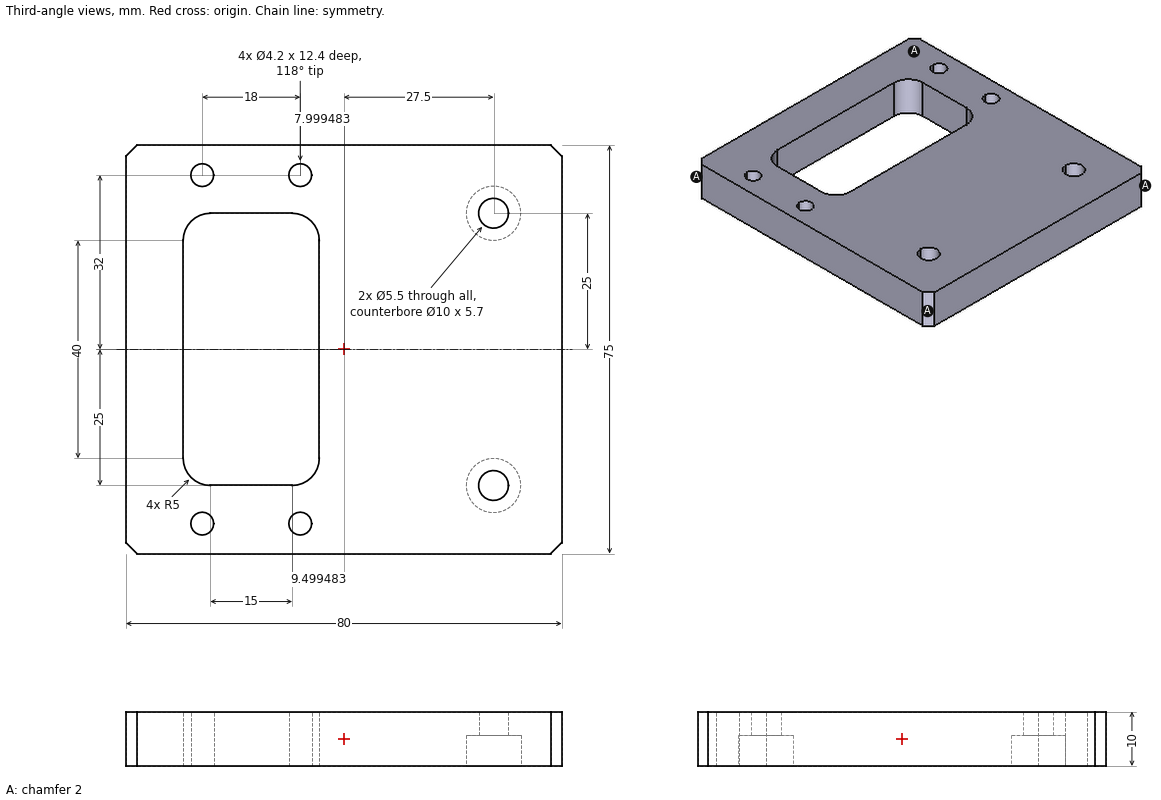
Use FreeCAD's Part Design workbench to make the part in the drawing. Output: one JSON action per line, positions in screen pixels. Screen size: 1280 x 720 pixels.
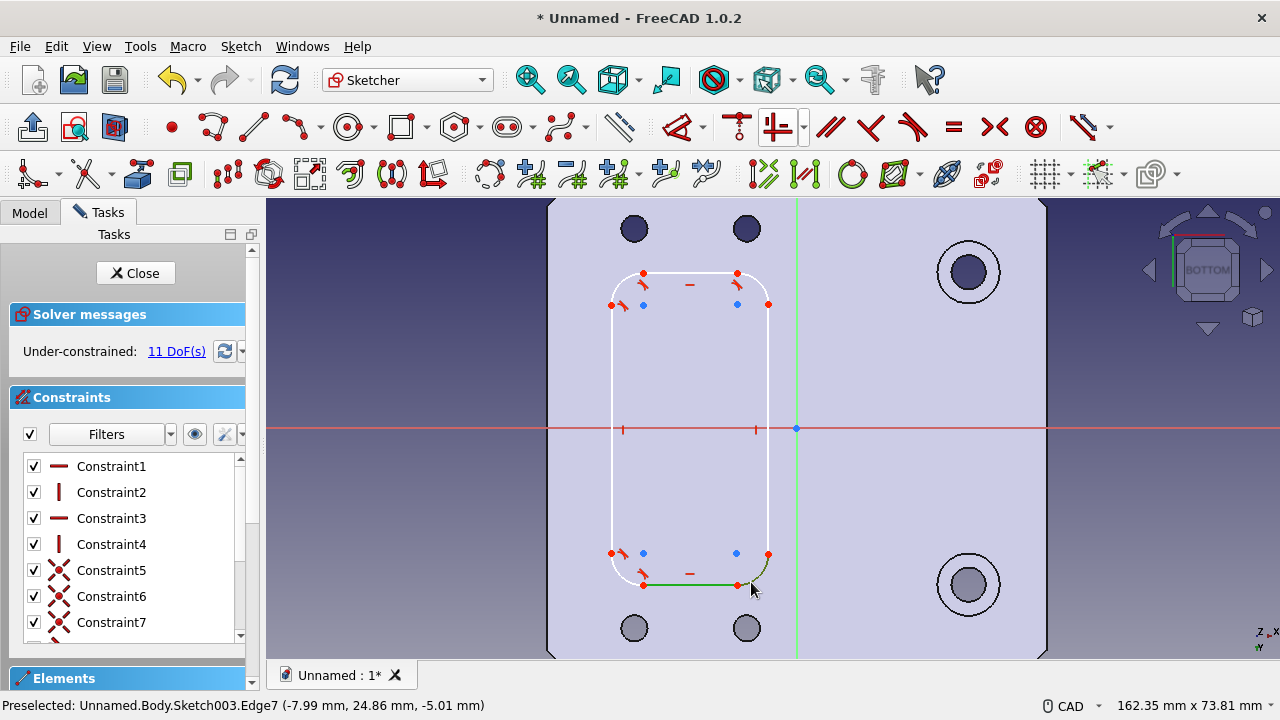
{"action": "key", "text": "t"}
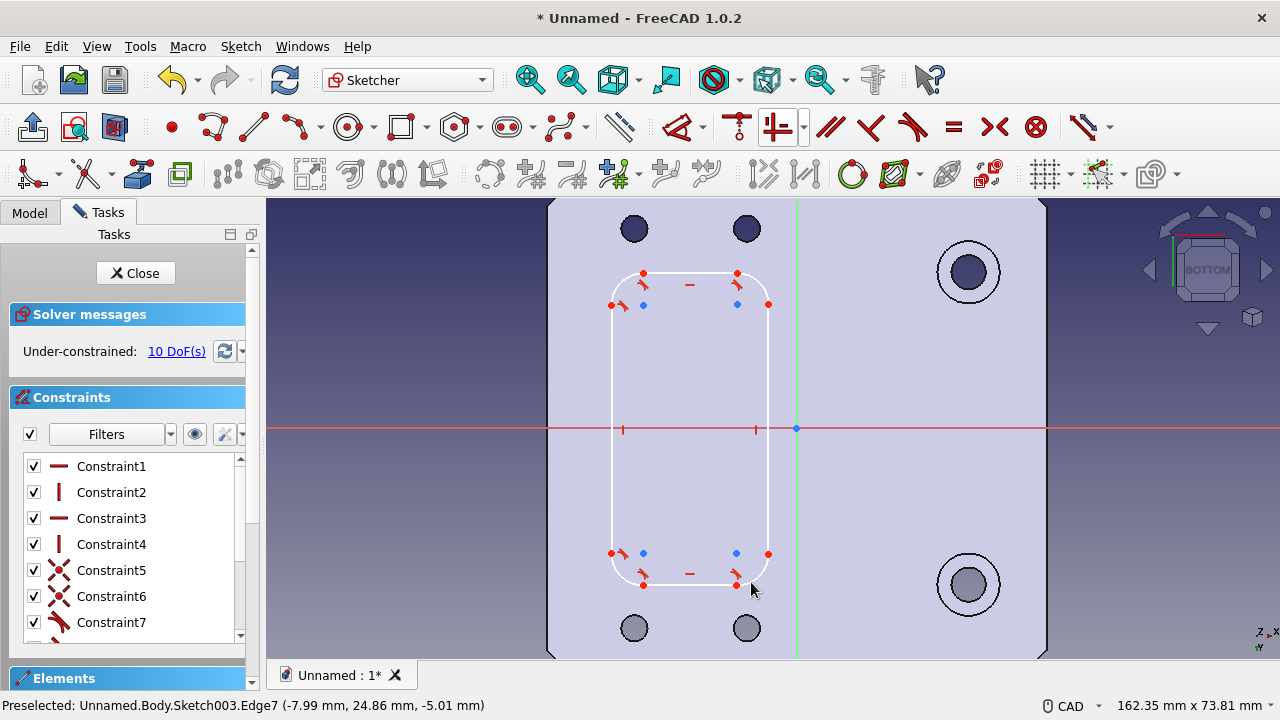
{"action": "left_click", "coordinate": [768, 479]}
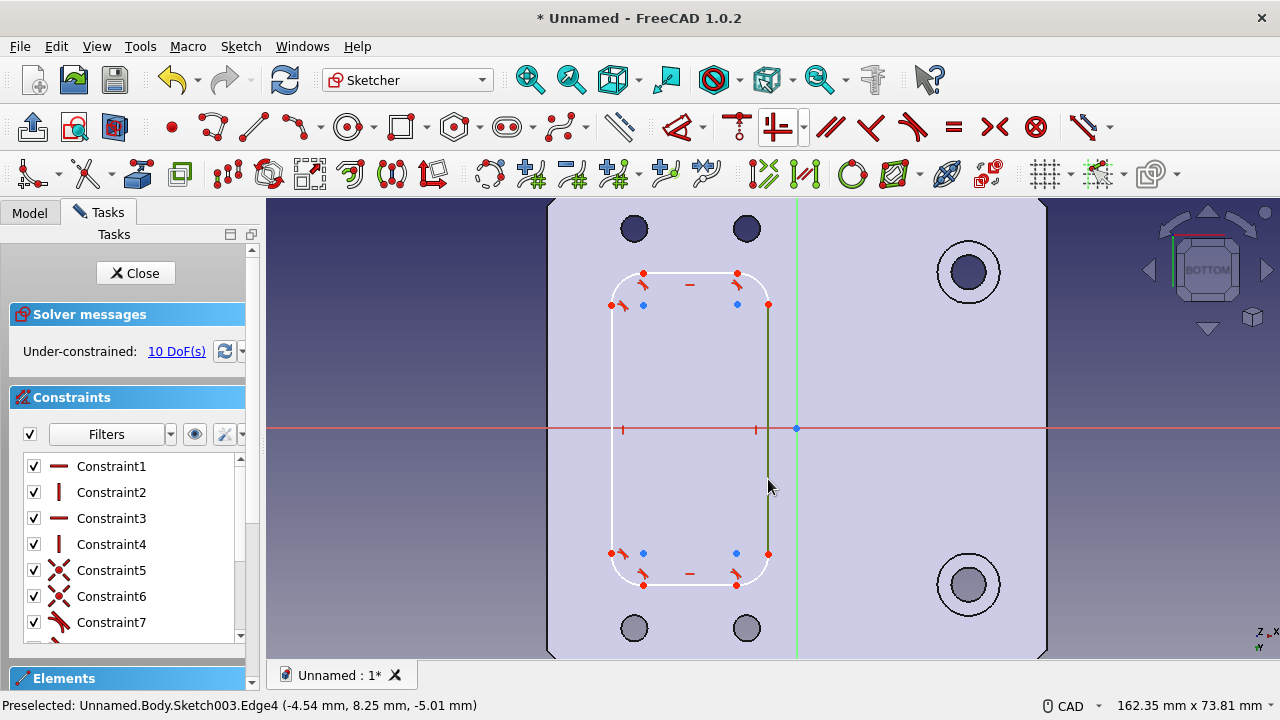
{"action": "left_click", "coordinate": [751, 582]}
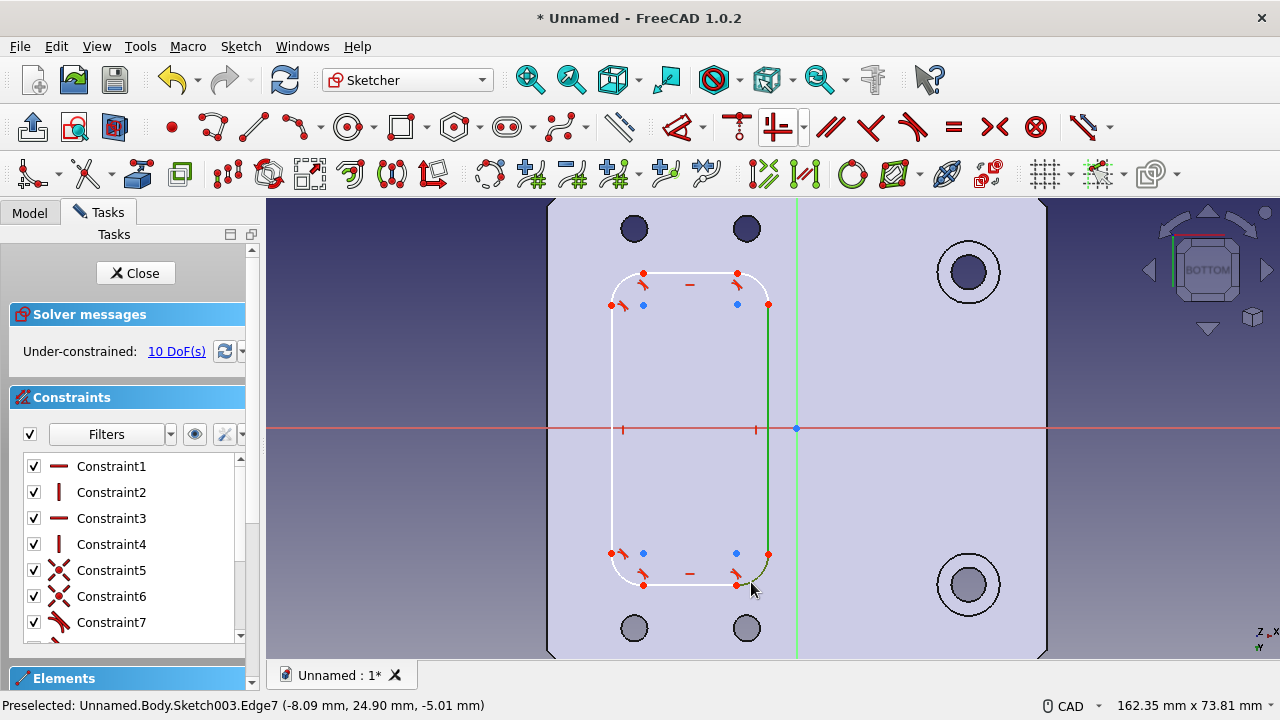
{"action": "key", "text": "t"}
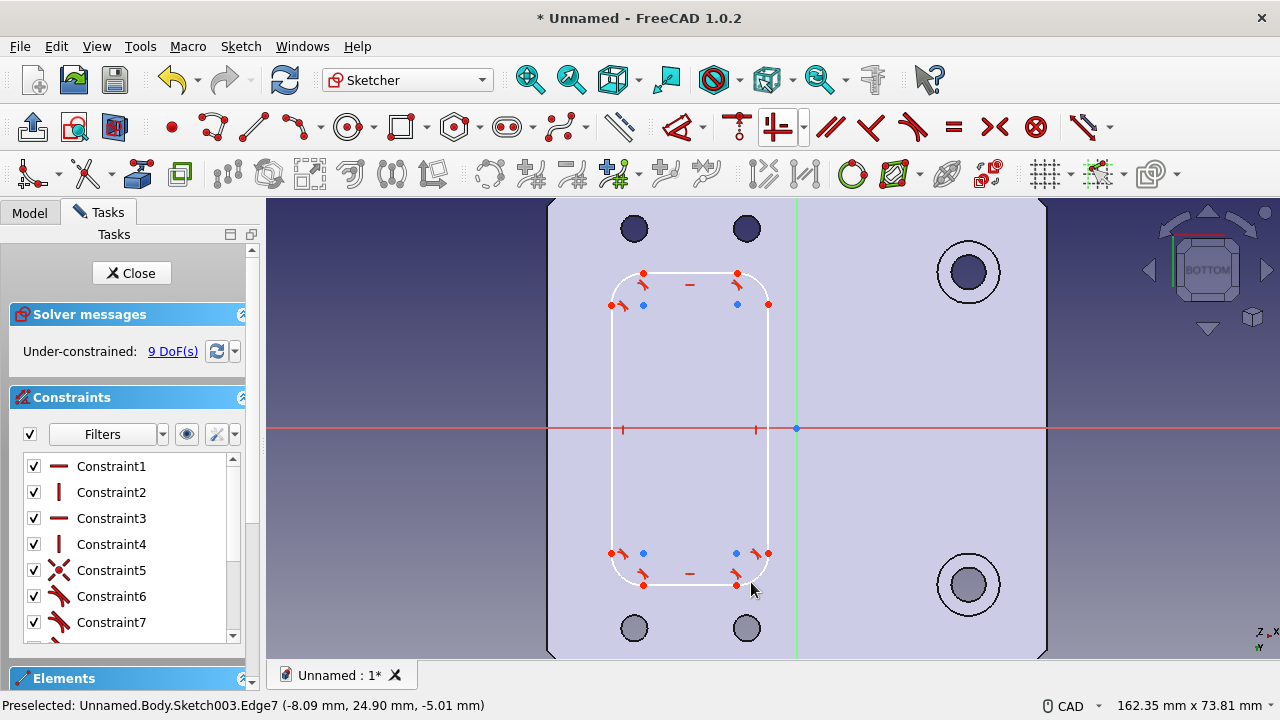
{"action": "left_click", "coordinate": [768, 479]}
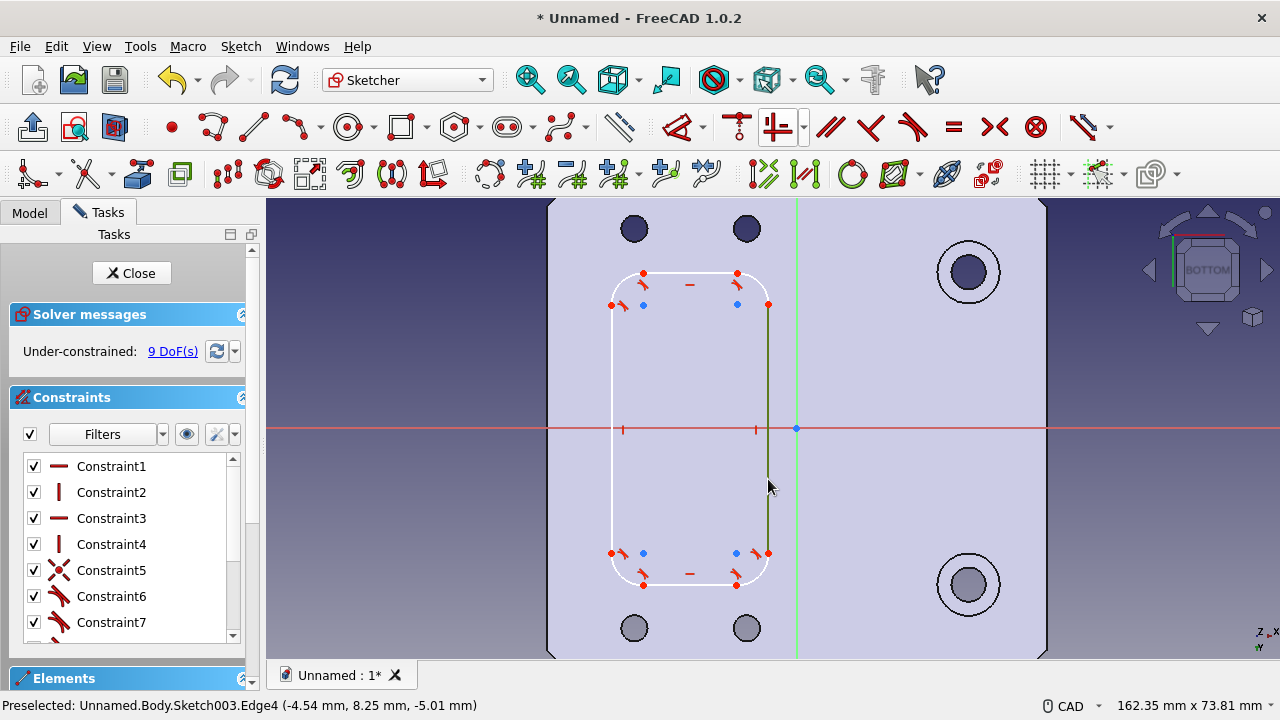
{"action": "left_click", "coordinate": [765, 290]}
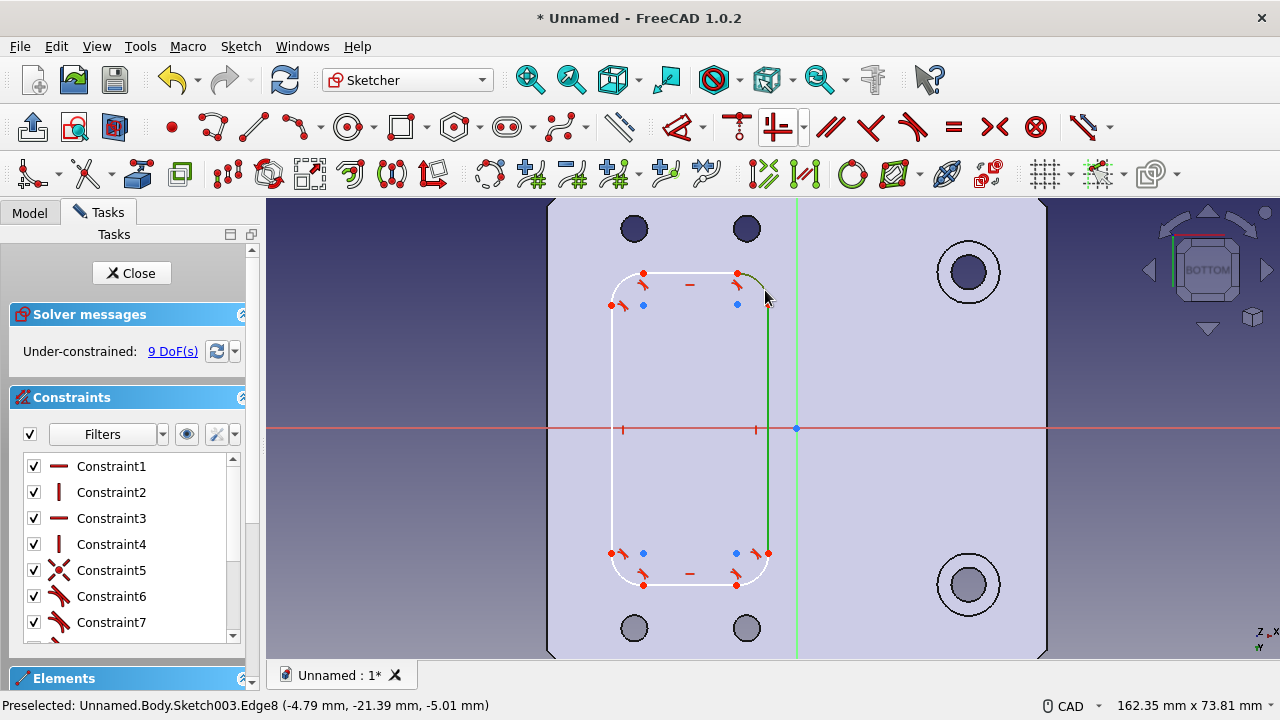
{"action": "key", "text": "t"}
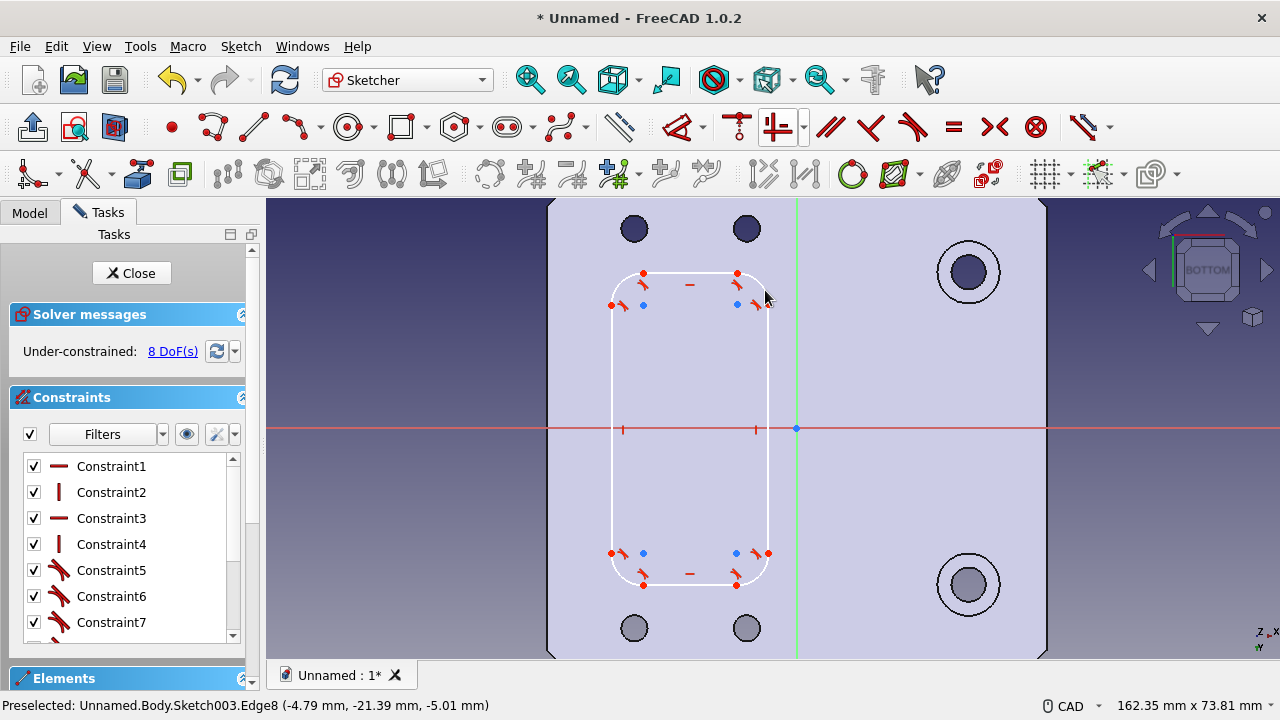
{"action": "left_click", "coordinate": [629, 277]}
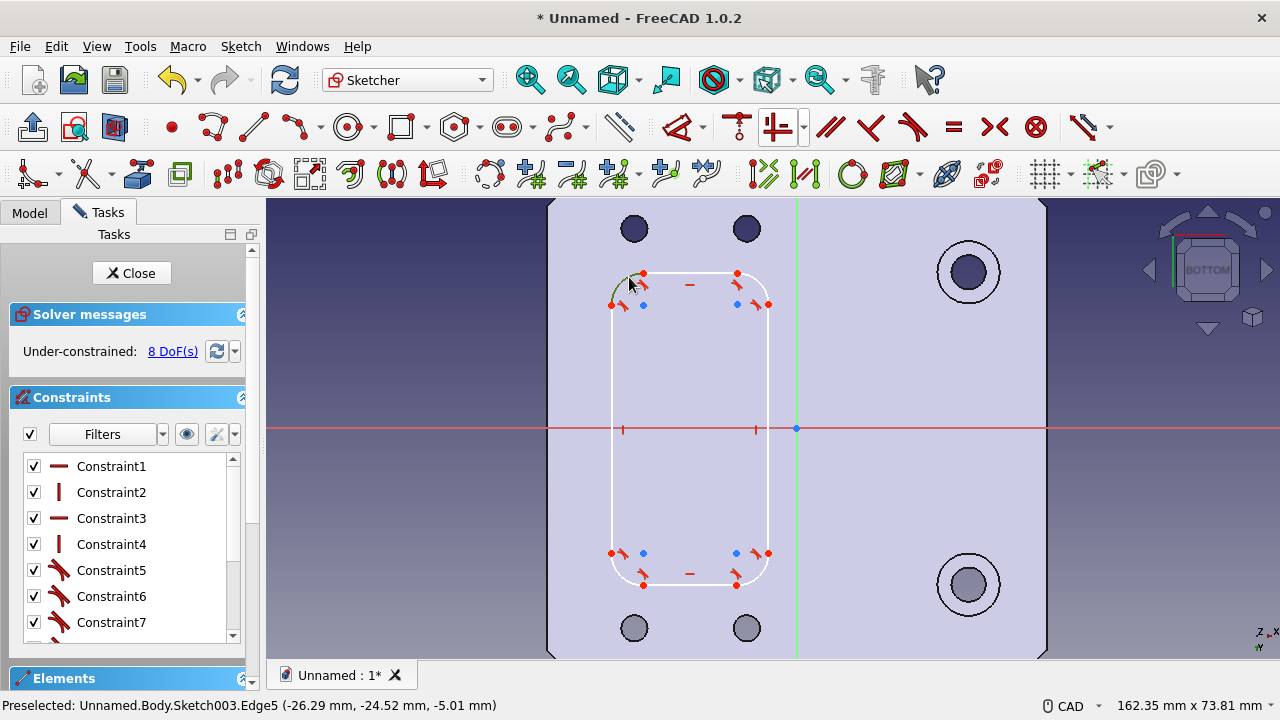
{"action": "left_click", "coordinate": [615, 568]}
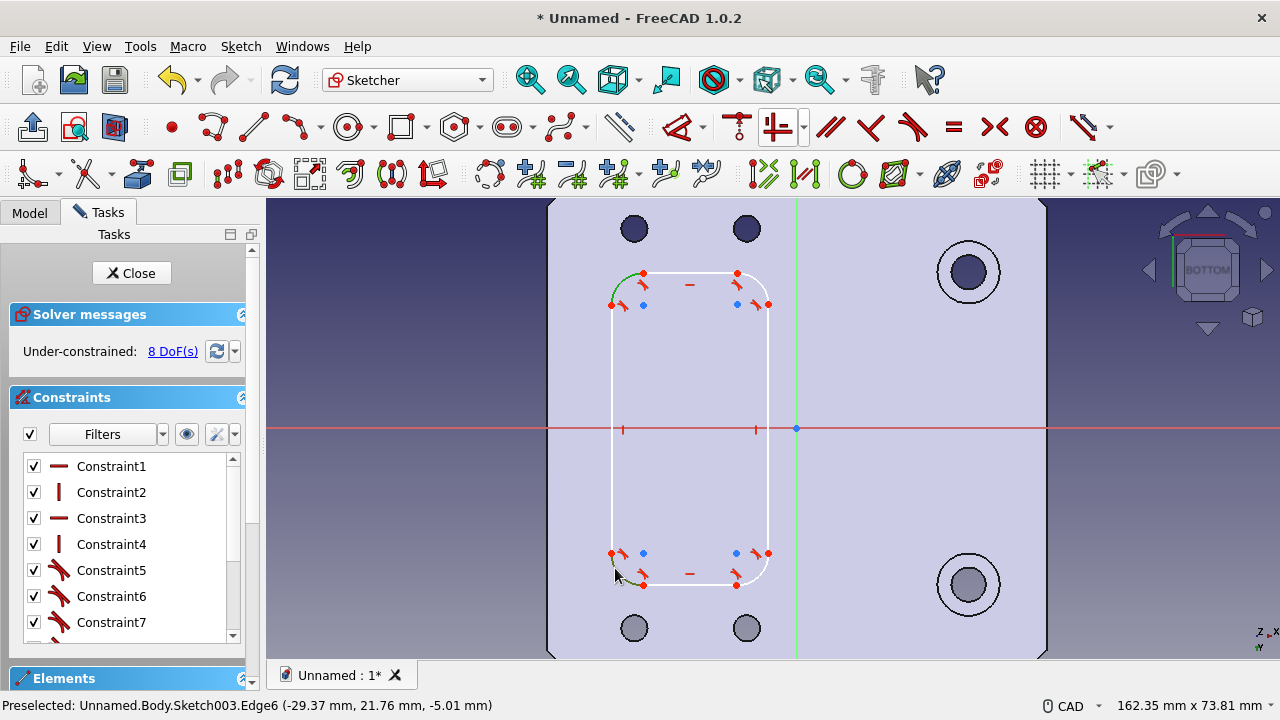
{"action": "left_click", "coordinate": [751, 582]}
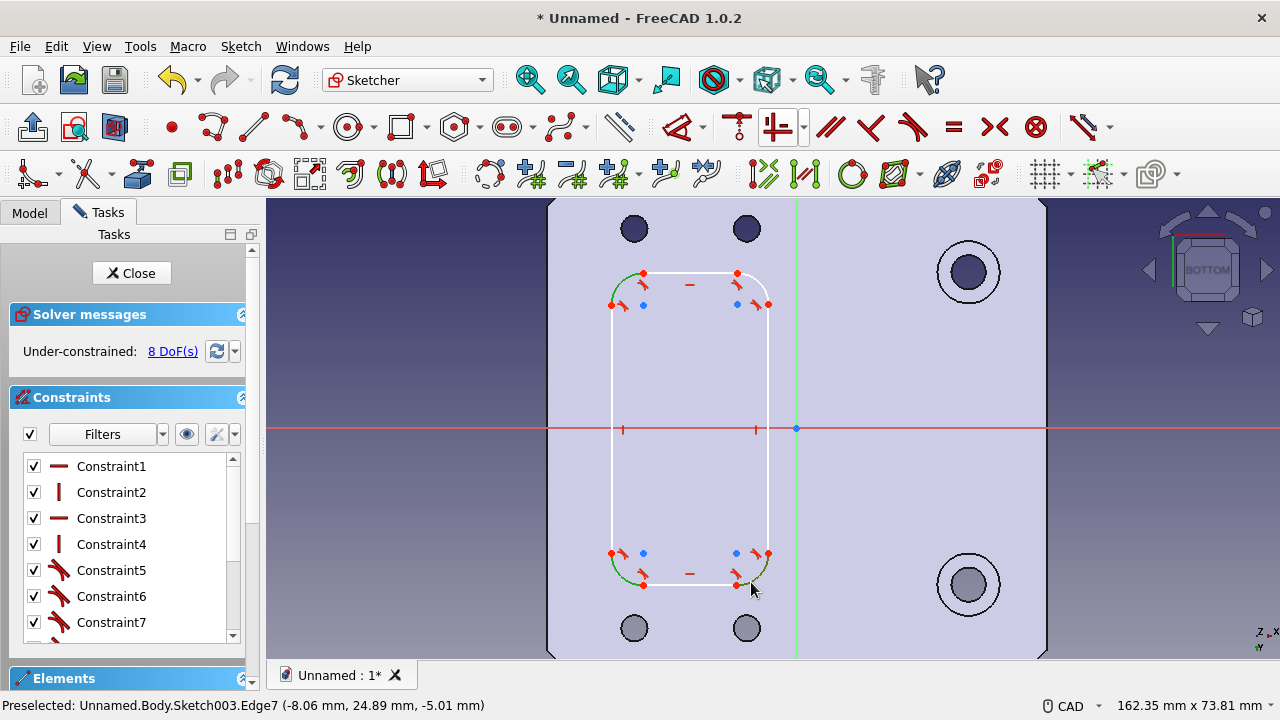
{"action": "left_click", "coordinate": [765, 290]}